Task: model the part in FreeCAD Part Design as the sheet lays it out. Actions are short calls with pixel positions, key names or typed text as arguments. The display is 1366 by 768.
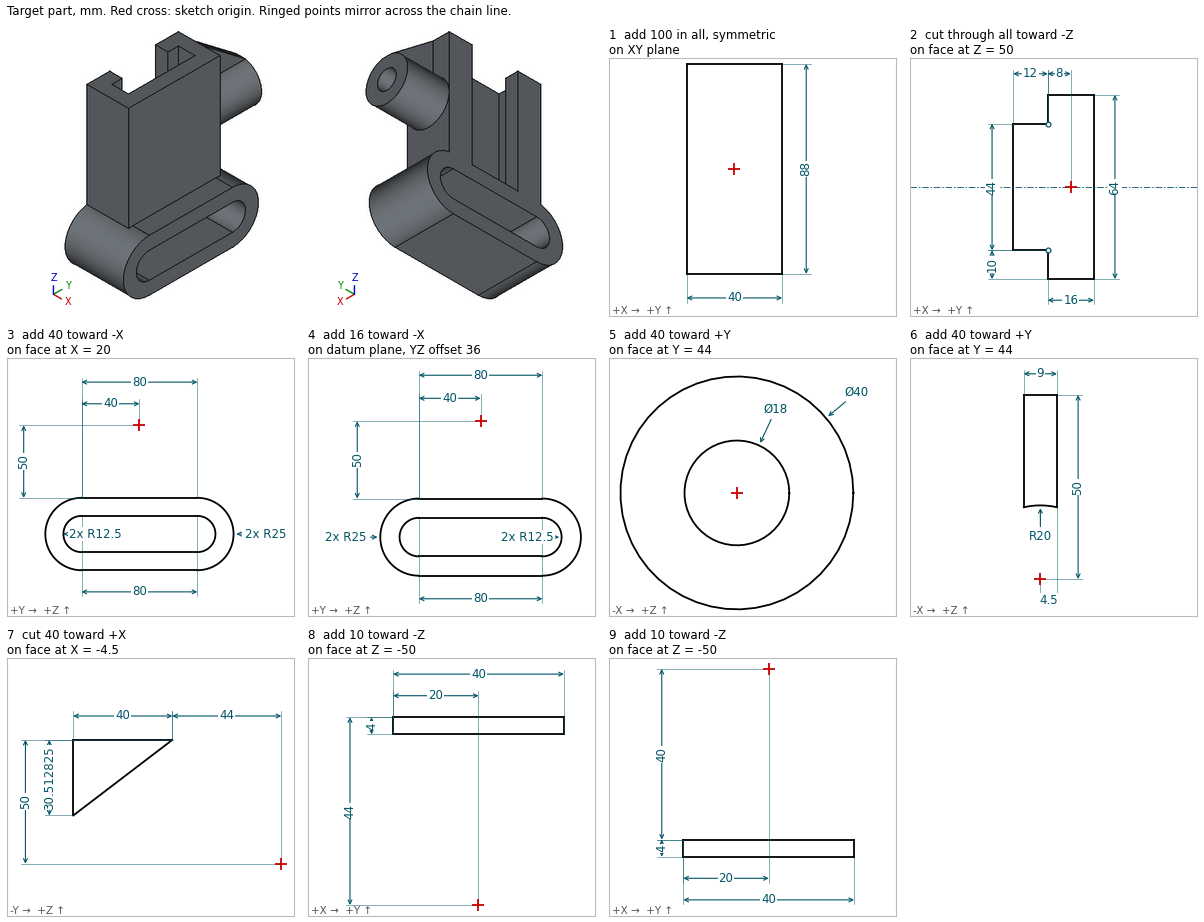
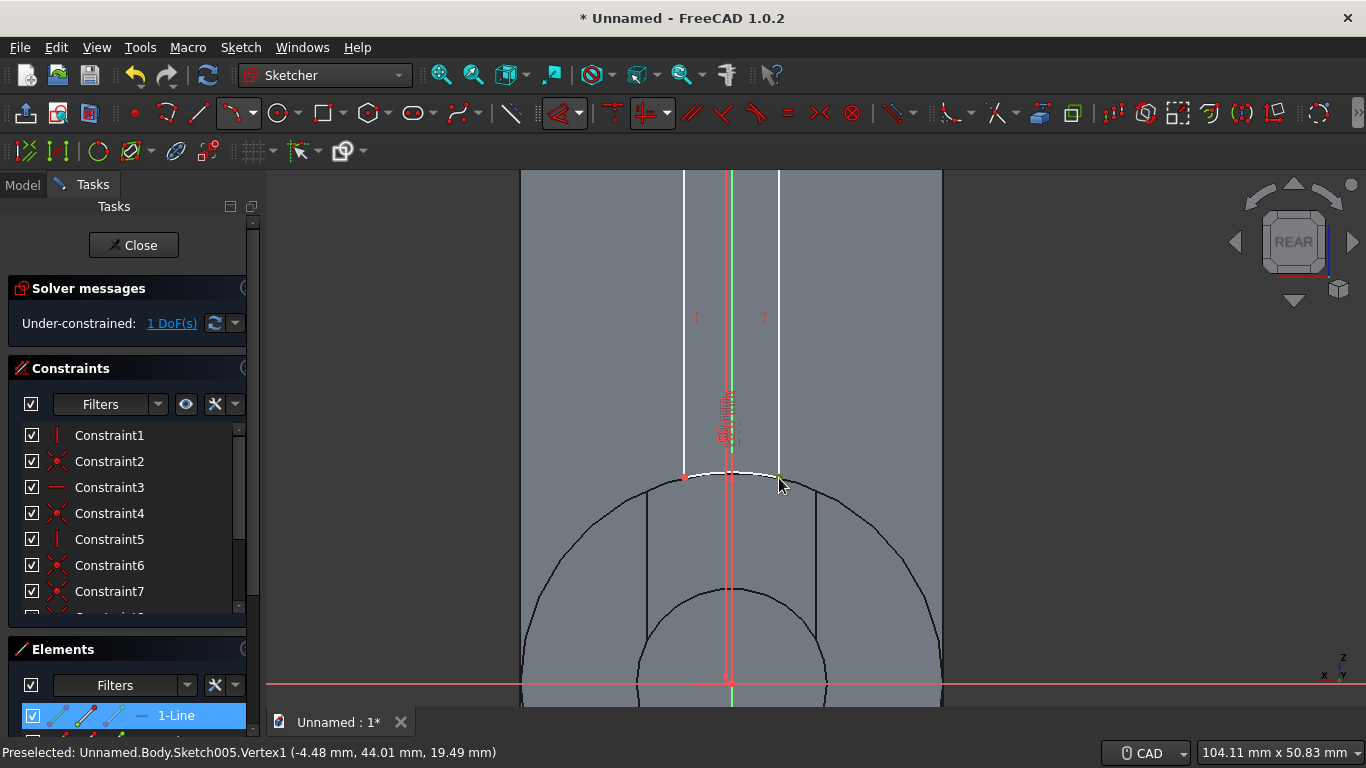
key(l)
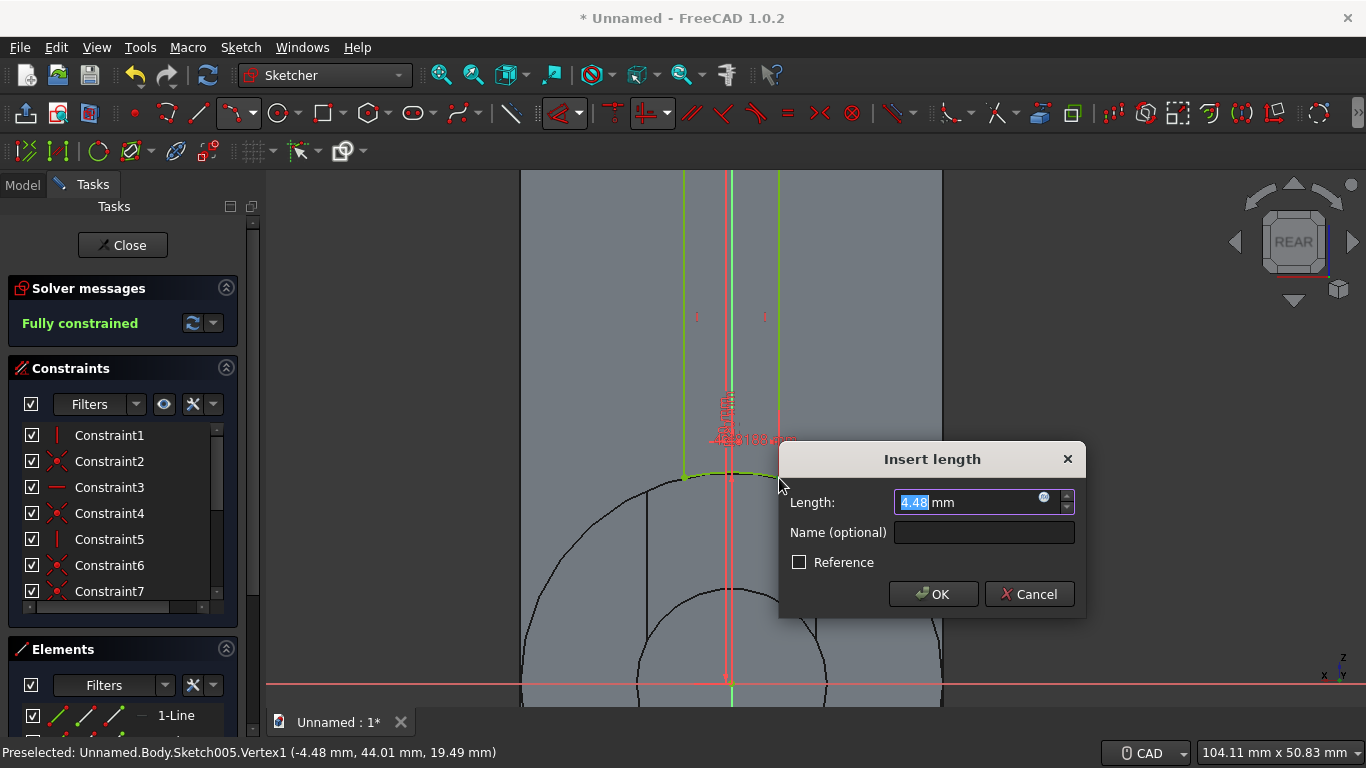
text(4.5)
key(Return)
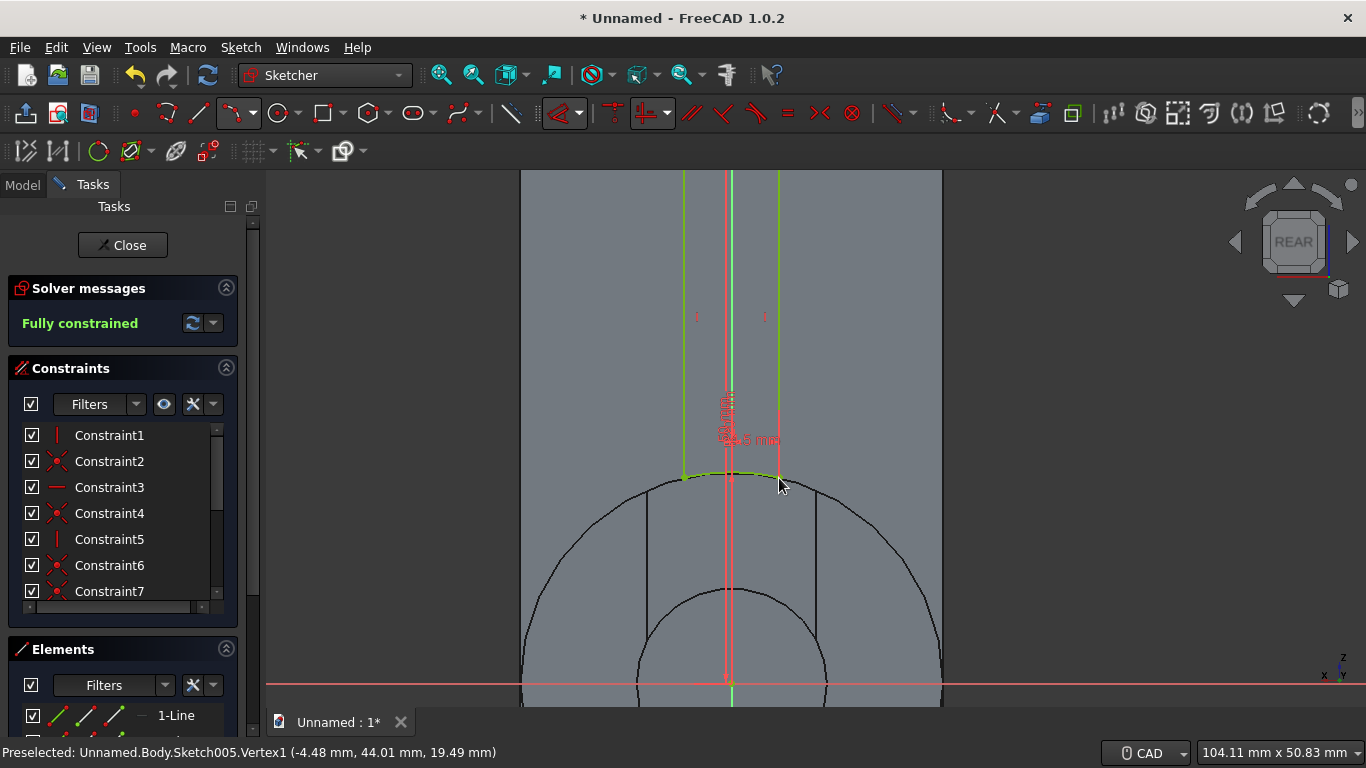
click(123, 245)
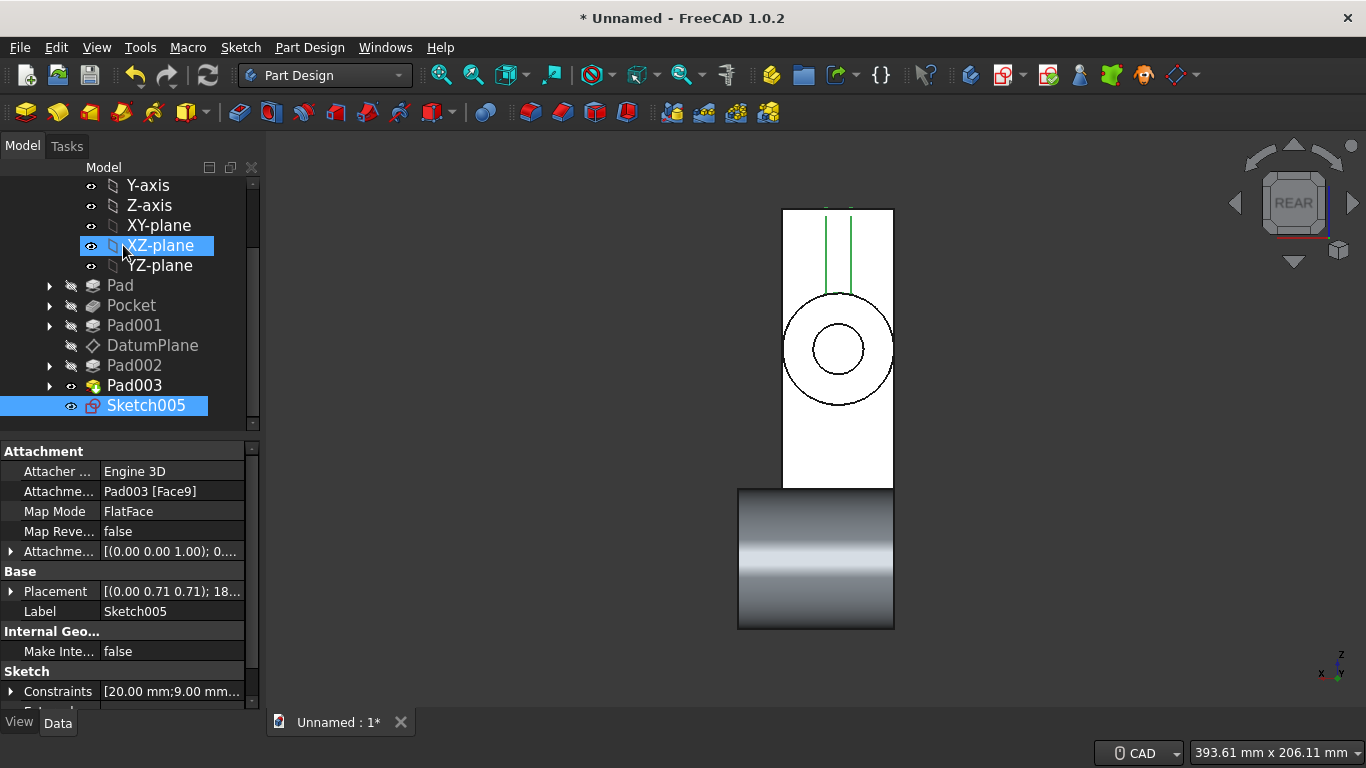
click(26, 112)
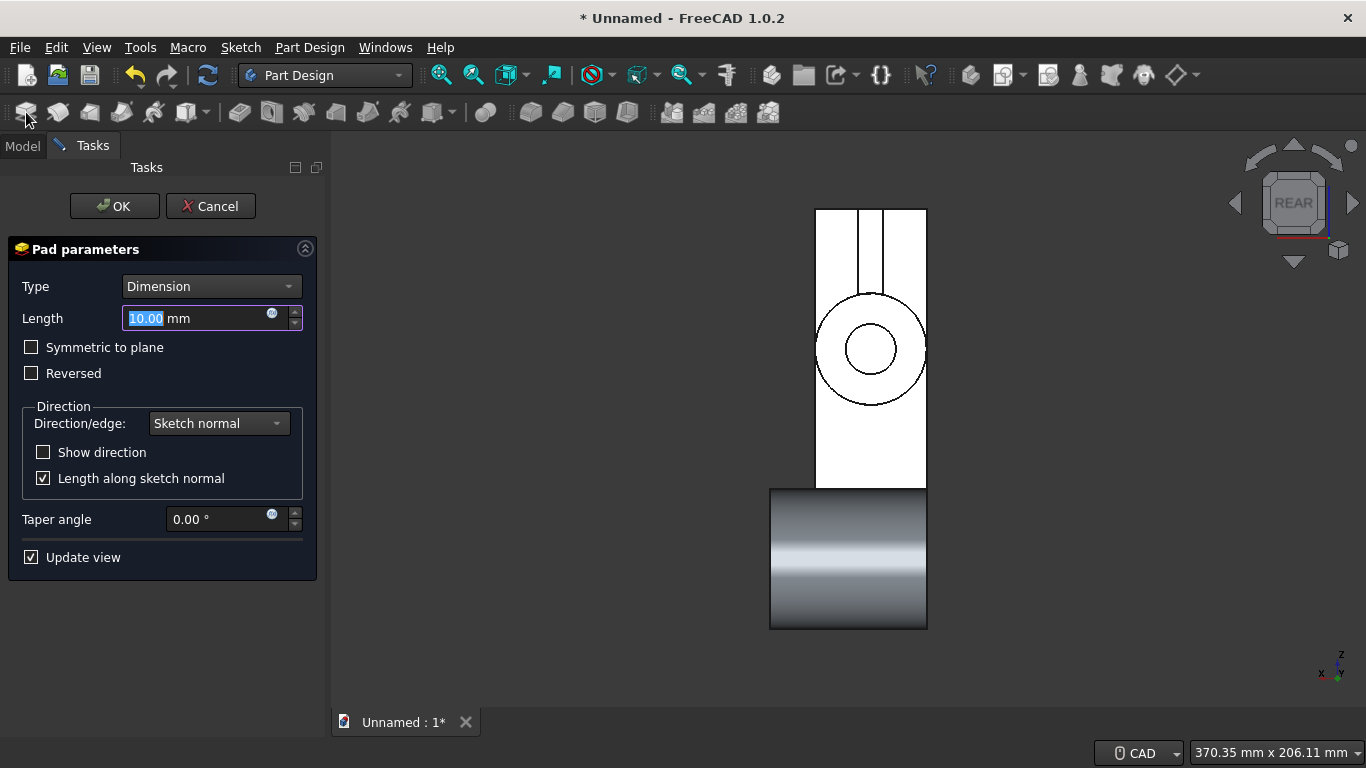
text(40)
key(Tab)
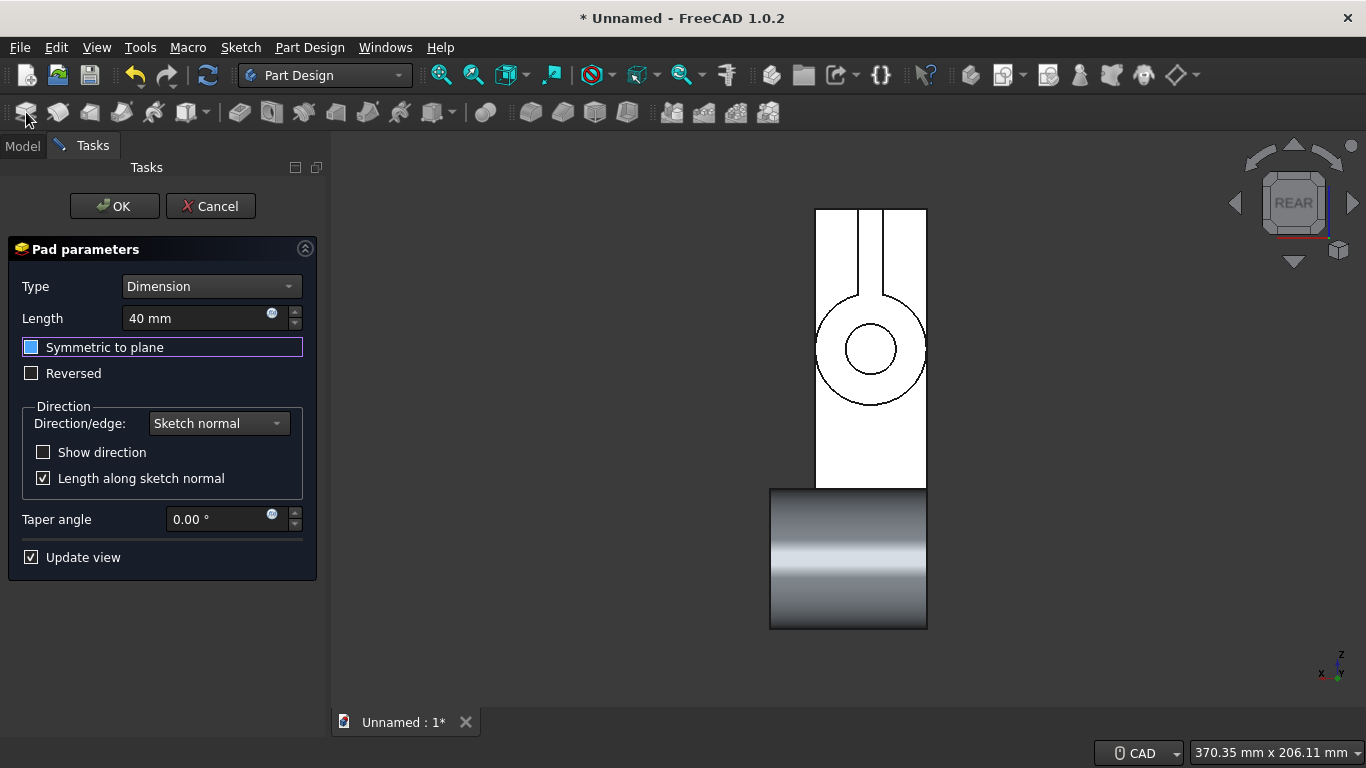
click(115, 206)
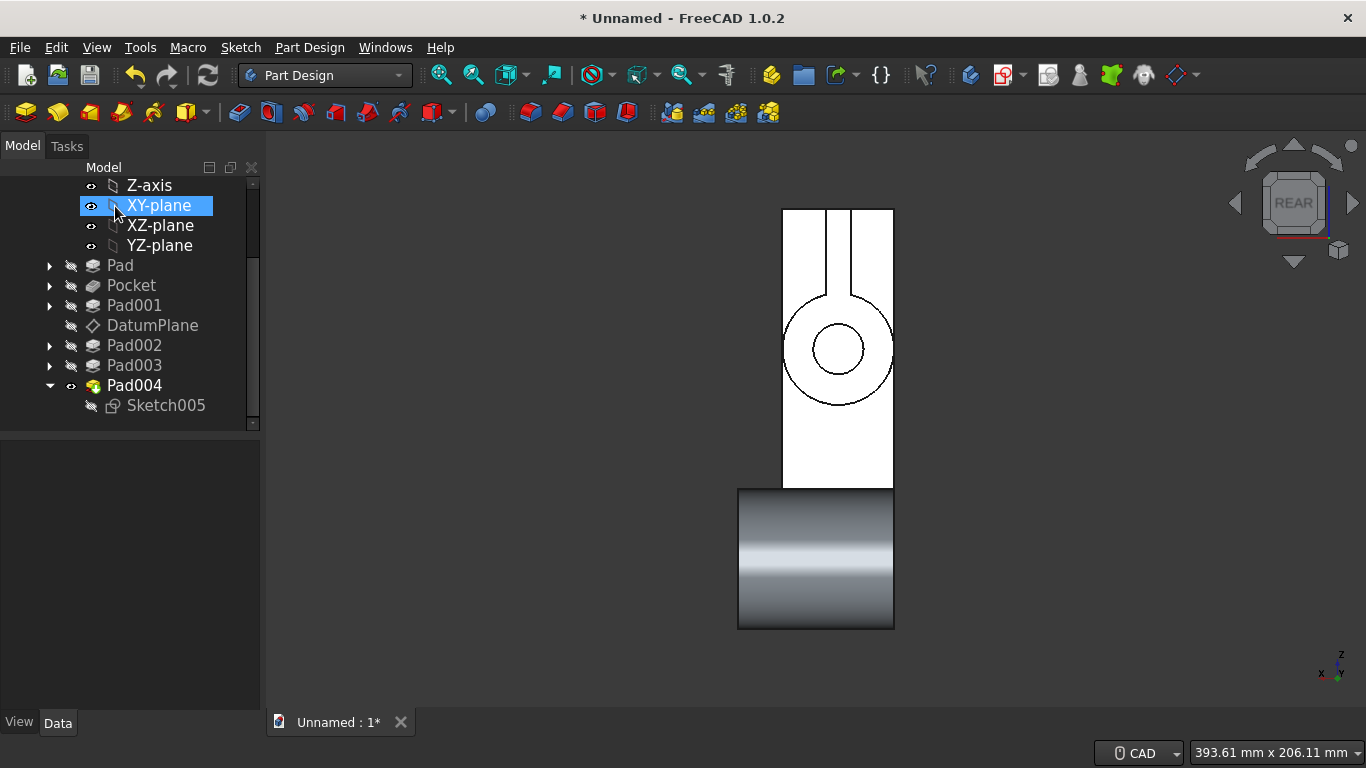
key(6)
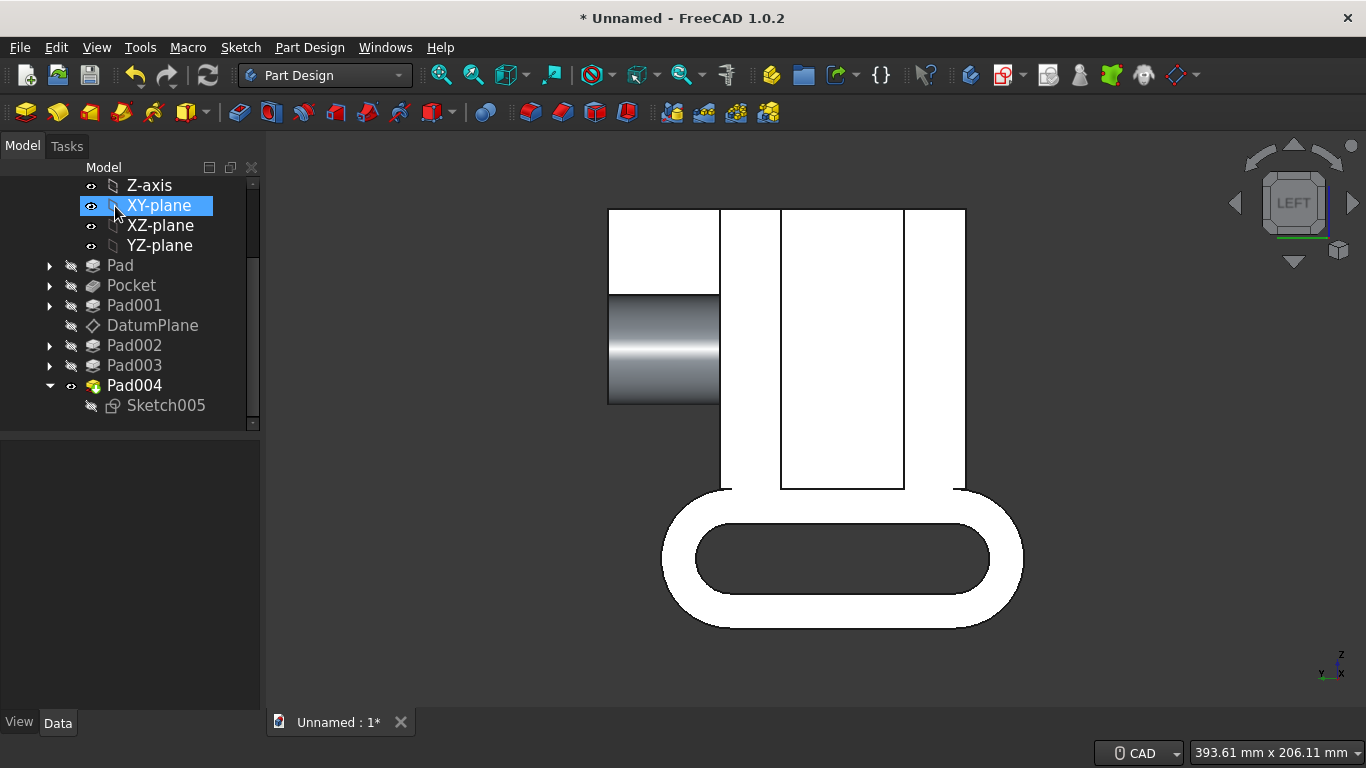
click(664, 251)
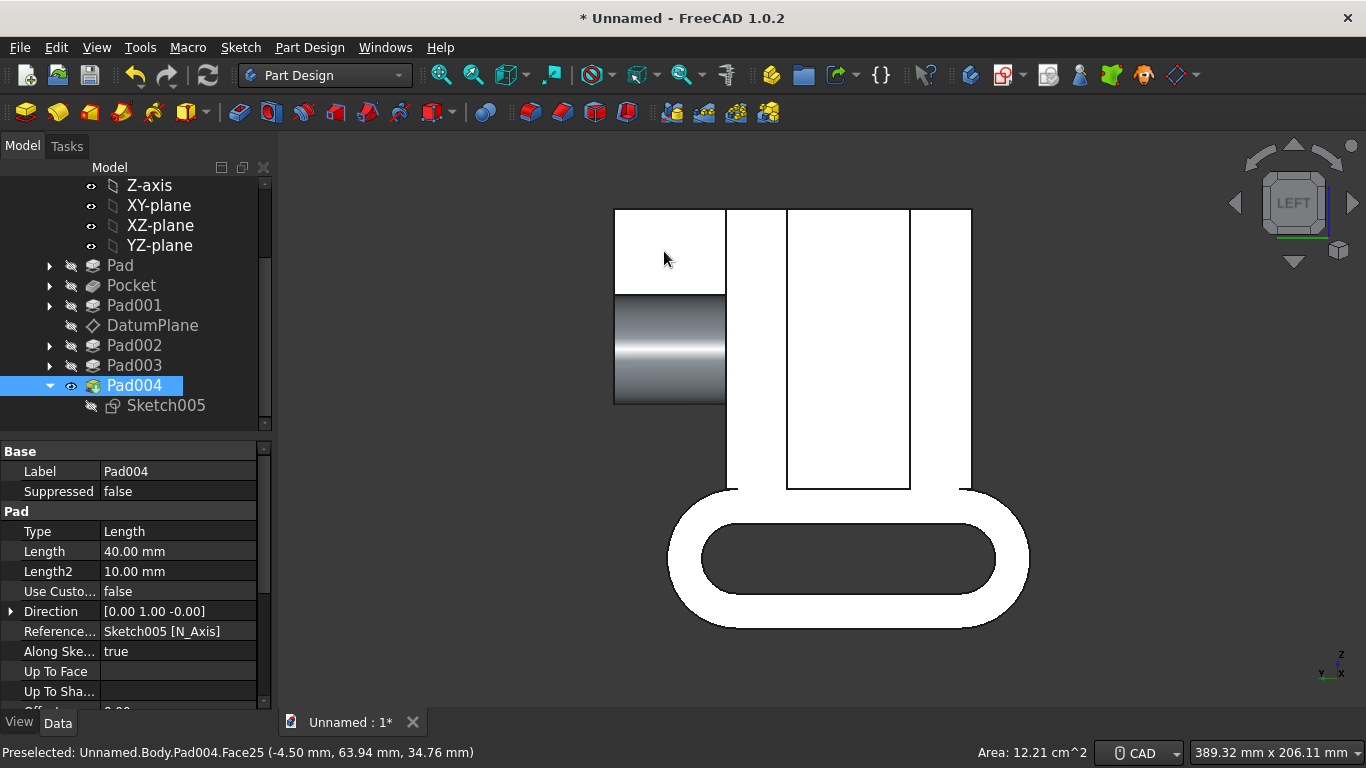
click(1004, 76)